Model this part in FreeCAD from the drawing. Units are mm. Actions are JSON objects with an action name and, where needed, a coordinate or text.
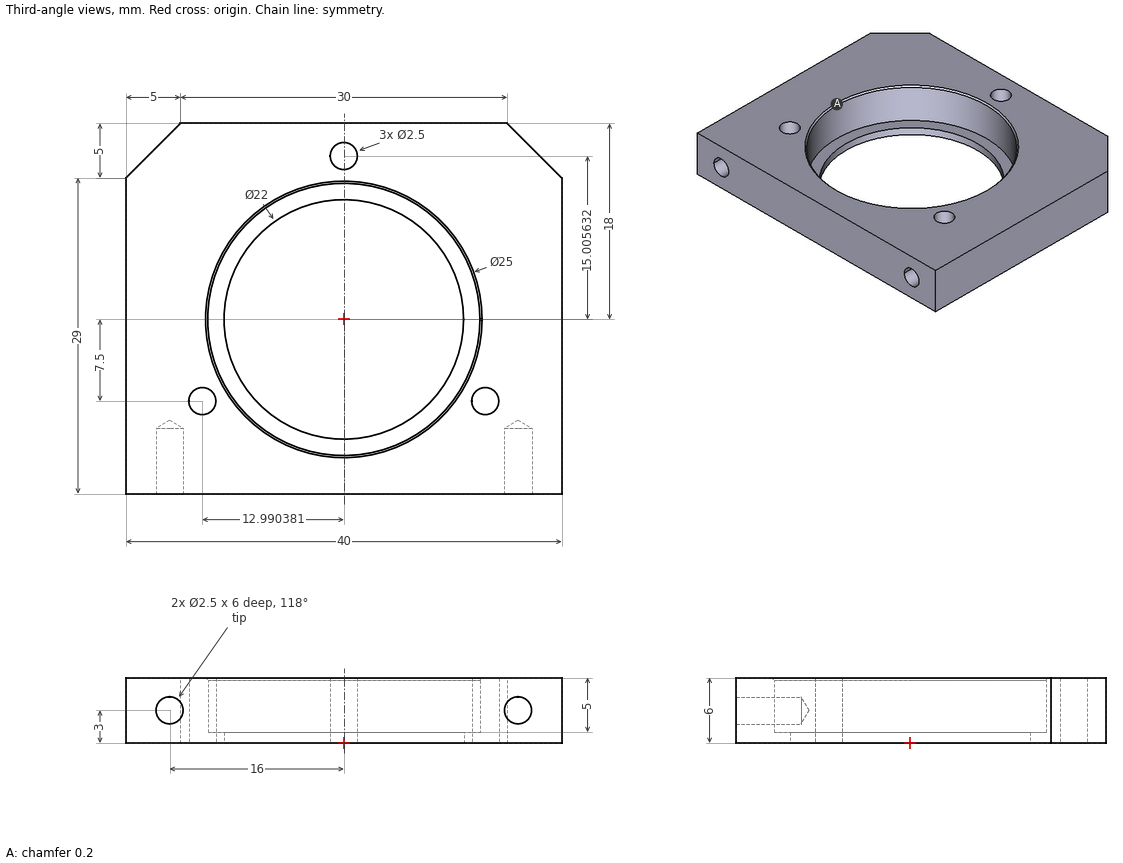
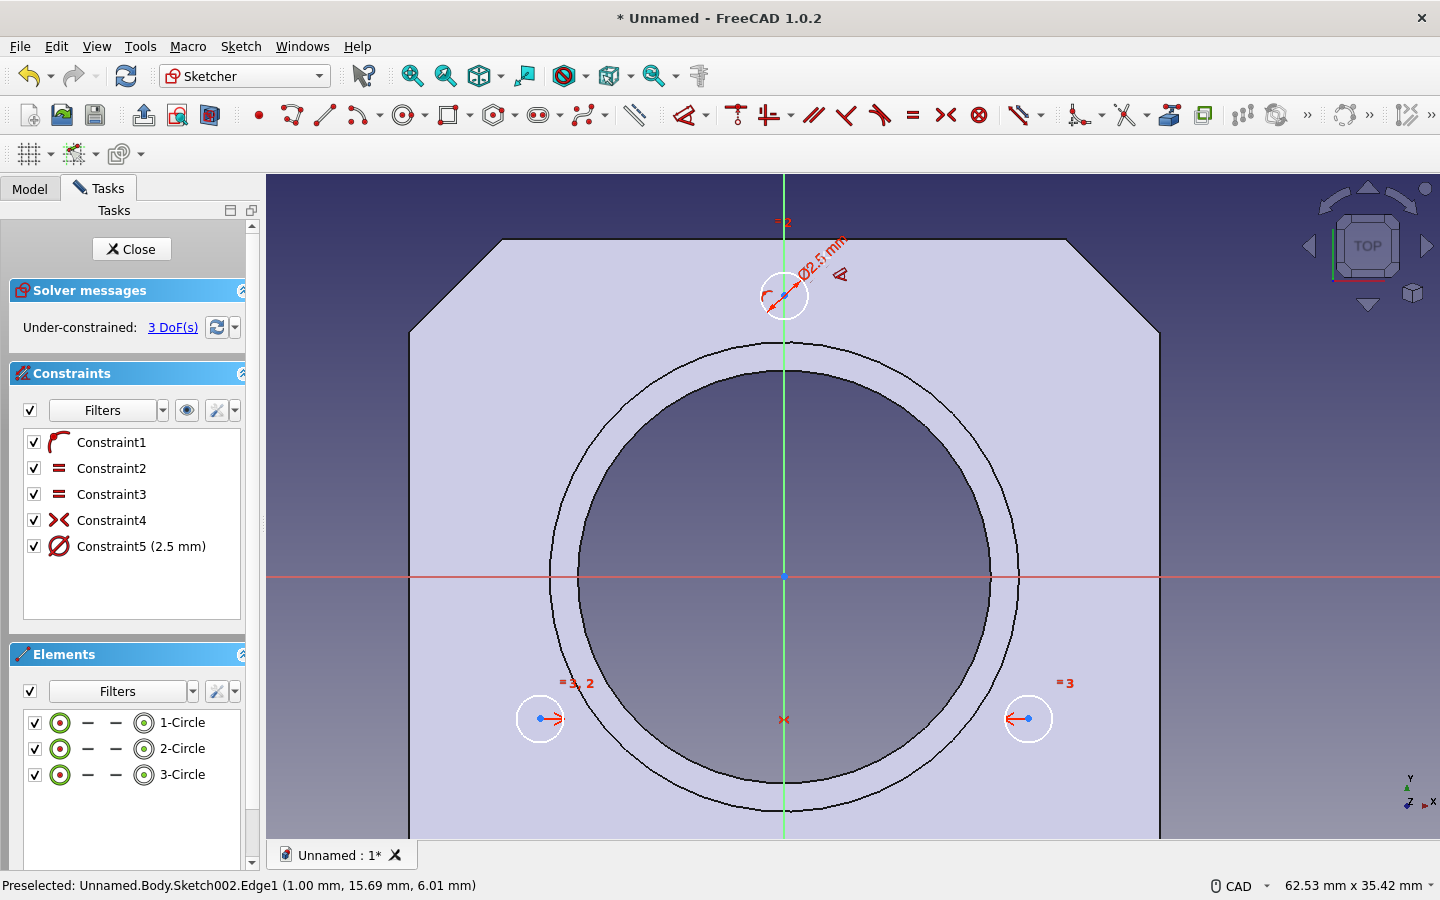
{"action": "left_click", "coordinate": [540, 719]}
{"action": "left_click", "coordinate": [506, 648]}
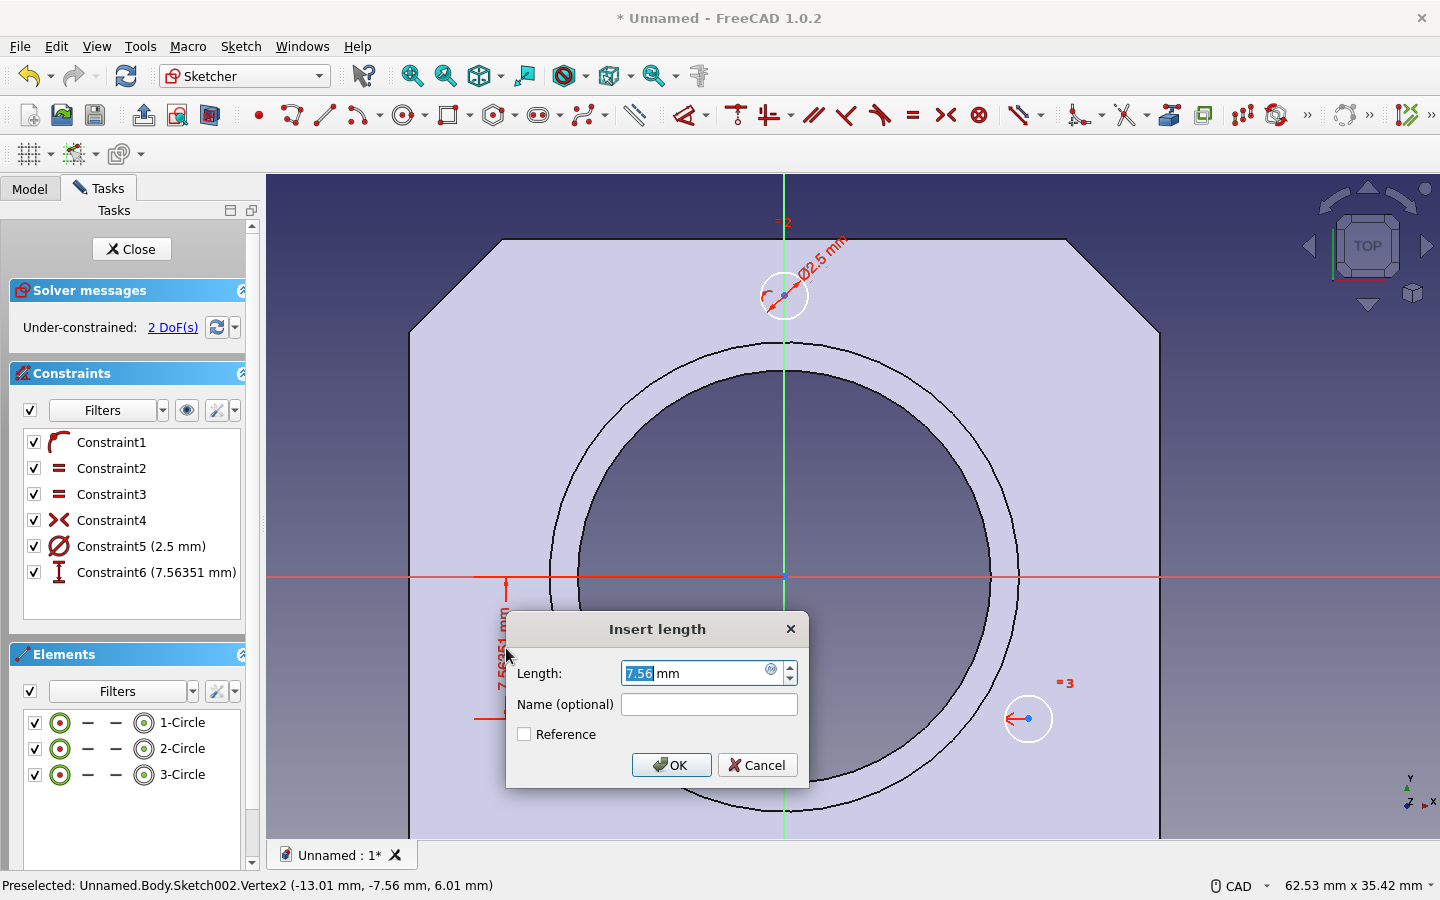
{"action": "type", "text": "7.5"}
{"action": "key", "text": "Return"}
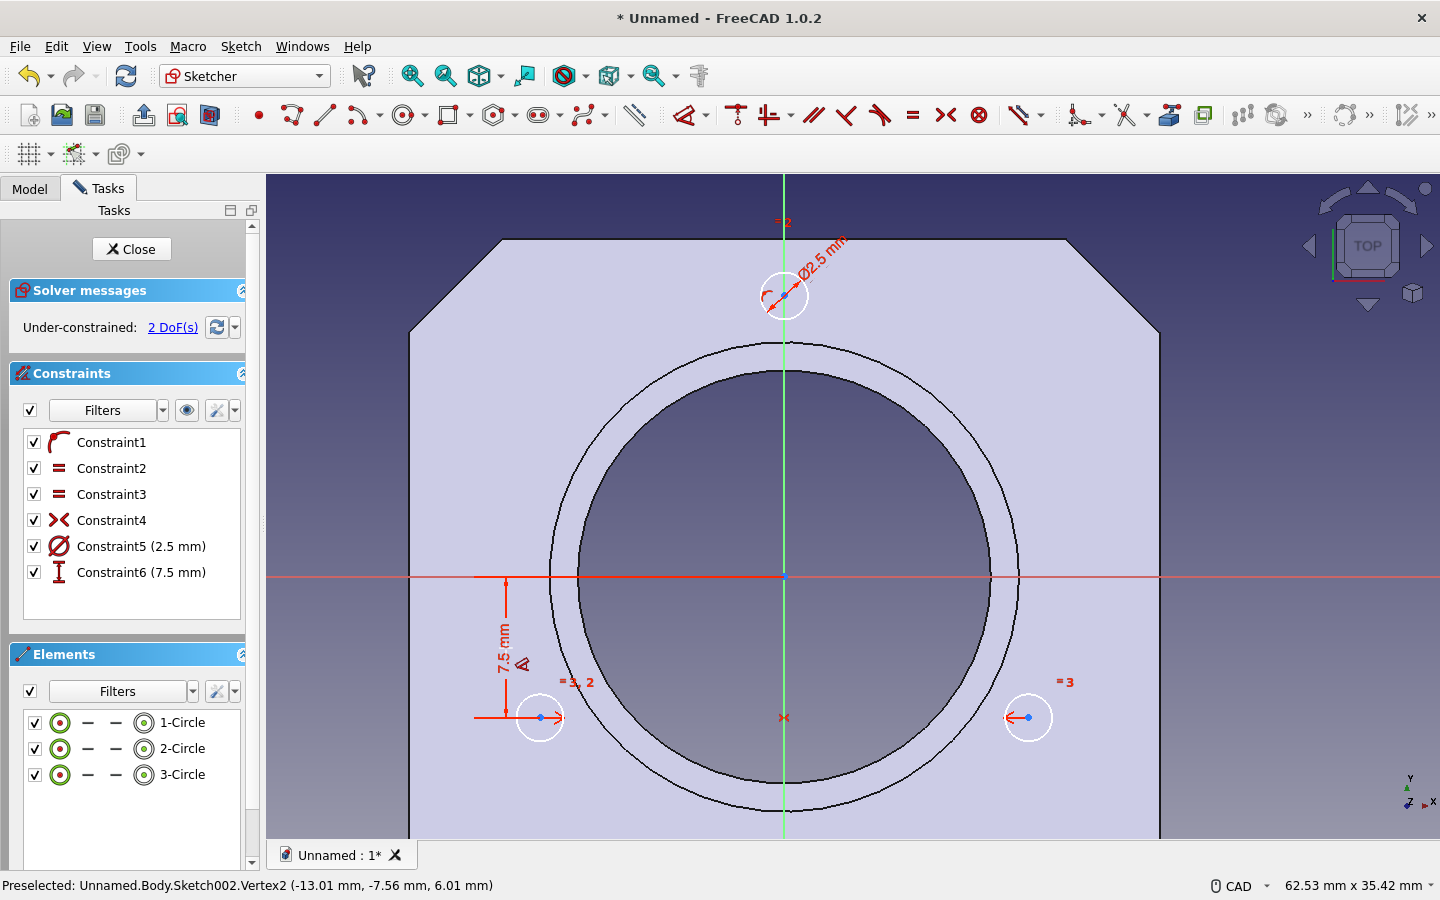
{"action": "left_click", "coordinate": [784, 296]}
{"action": "left_click", "coordinate": [818, 436]}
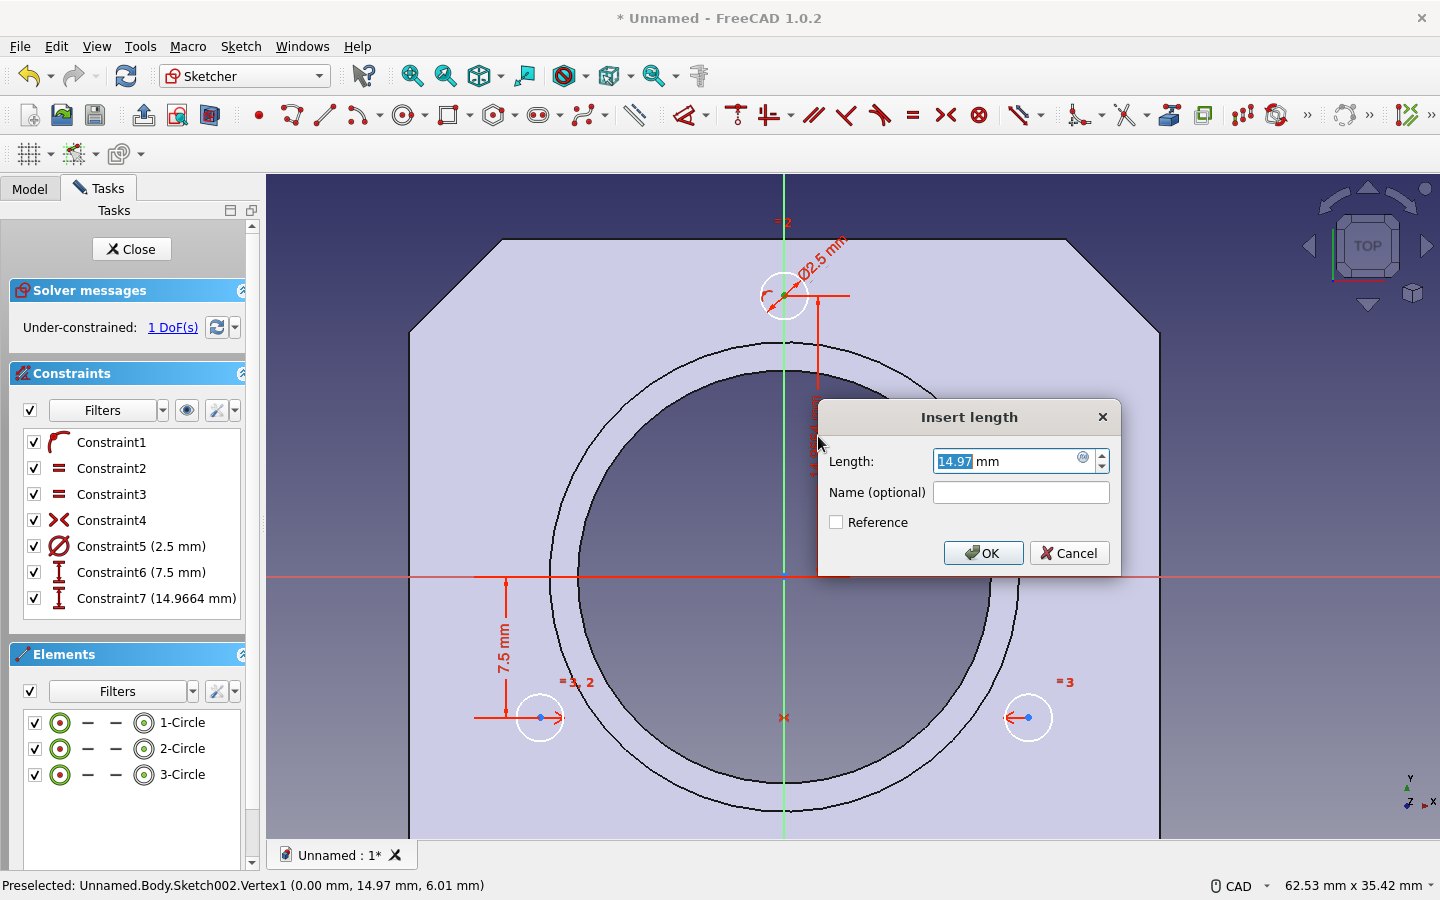
{"action": "type", "text": "15.005632"}
{"action": "key", "text": "Return"}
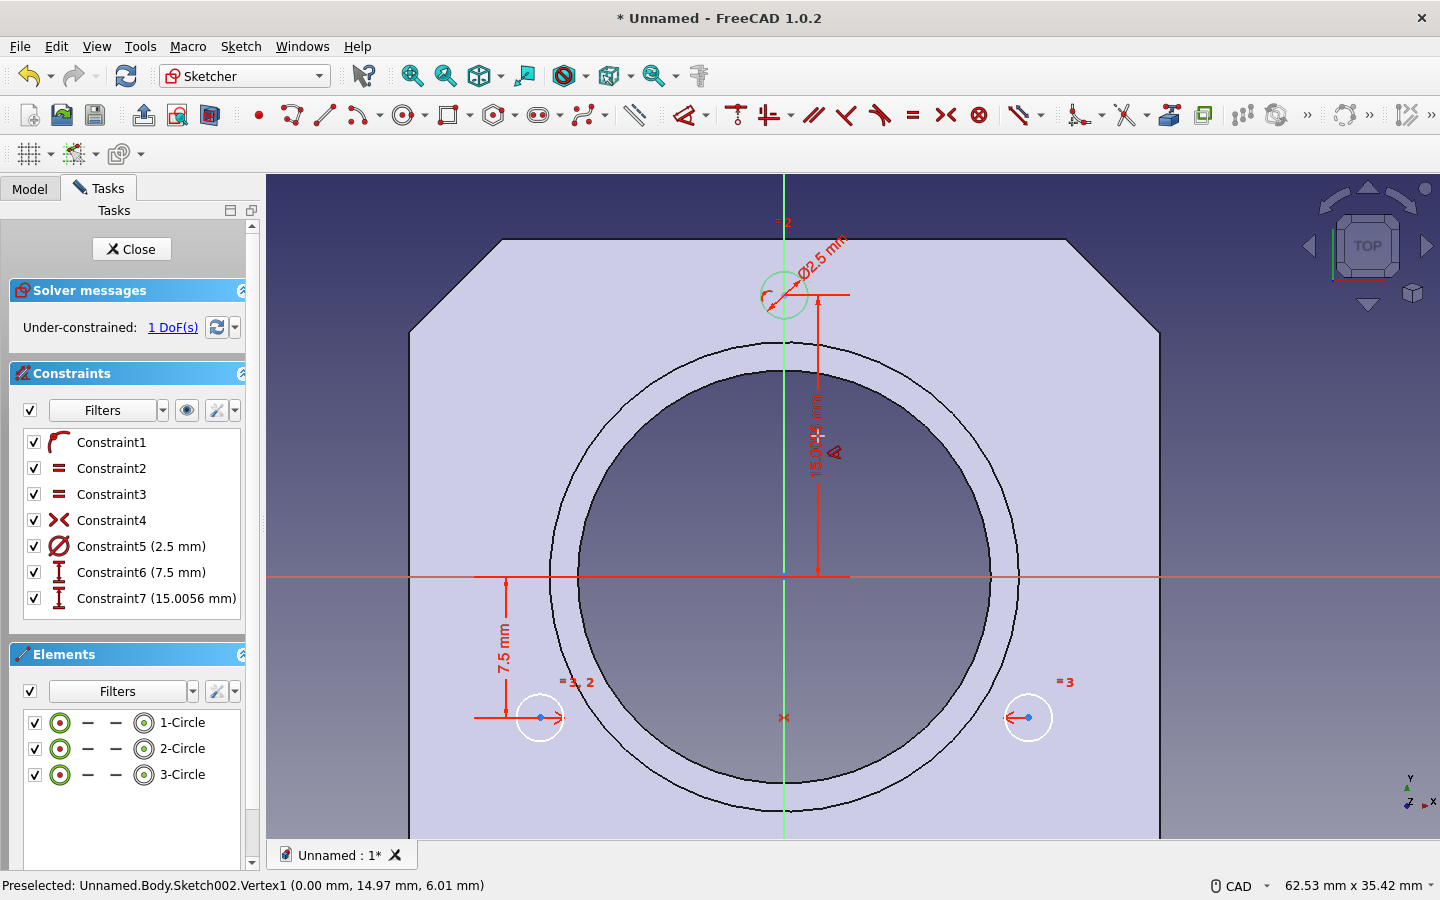
{"action": "left_click", "coordinate": [540, 718]}
{"action": "left_click", "coordinate": [662, 752]}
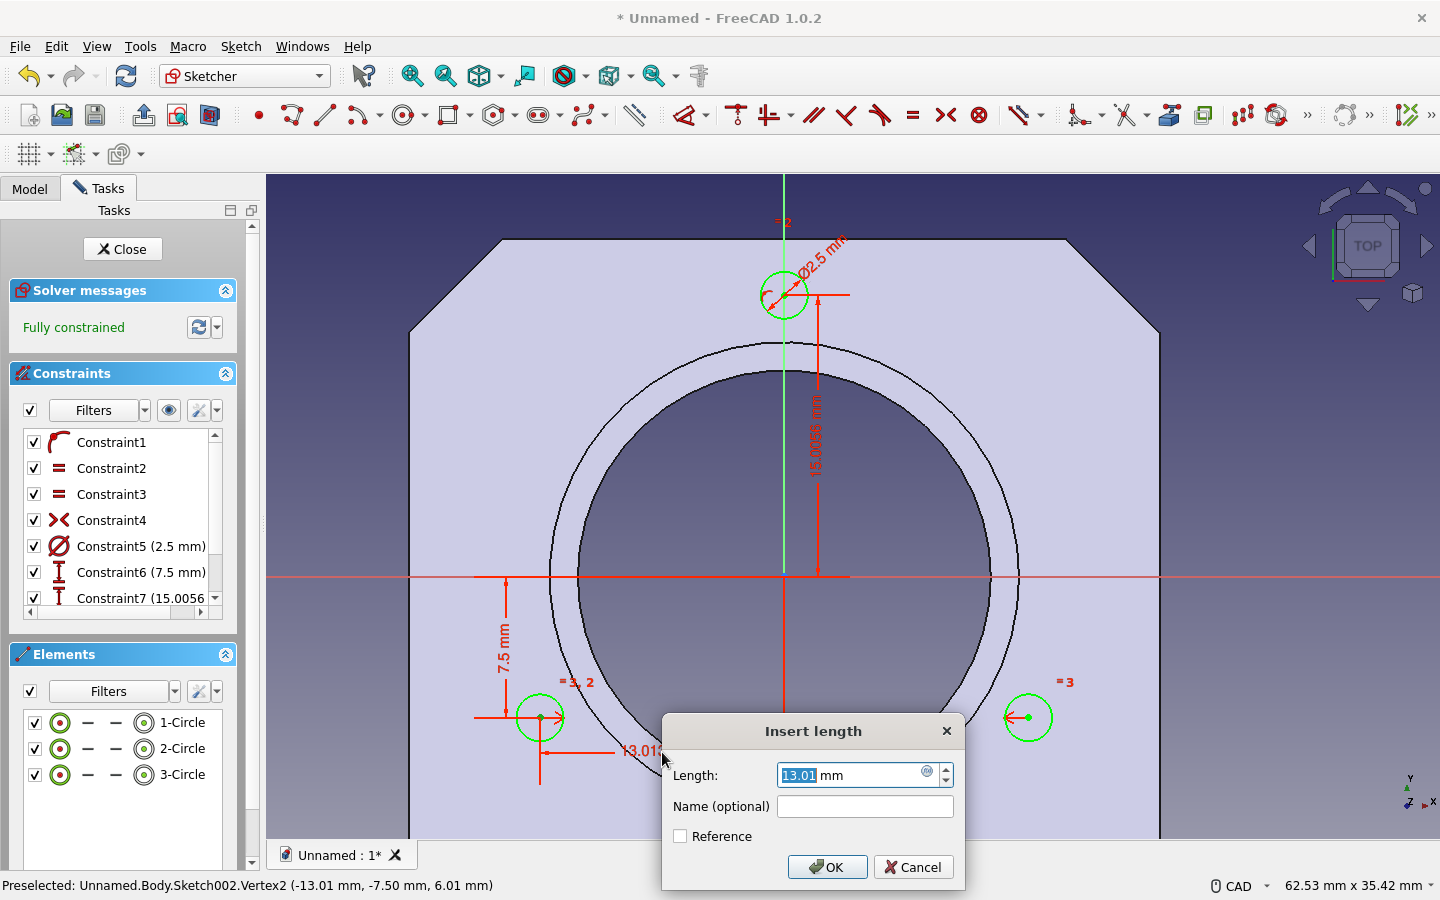
{"action": "type", "text": "12.990381"}
{"action": "key", "text": "Return"}
{"action": "key", "text": "Escape"}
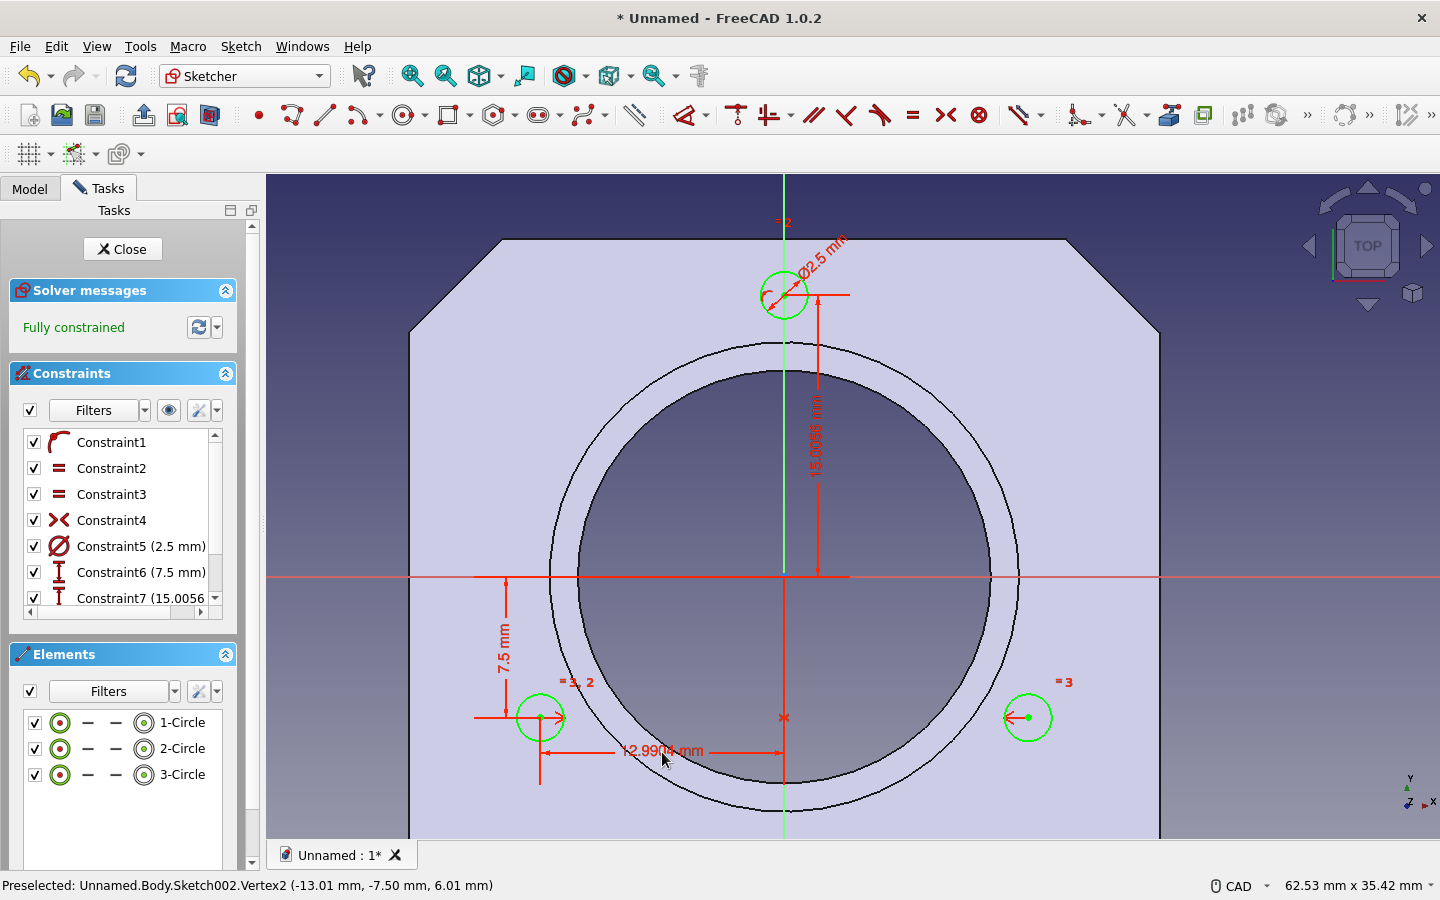
{"action": "left_click", "coordinate": [123, 249]}